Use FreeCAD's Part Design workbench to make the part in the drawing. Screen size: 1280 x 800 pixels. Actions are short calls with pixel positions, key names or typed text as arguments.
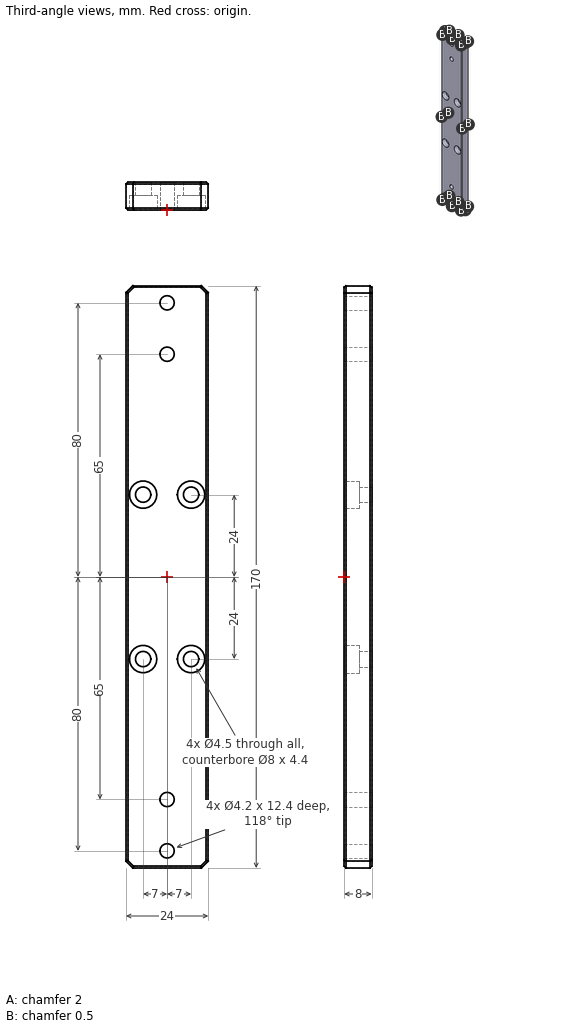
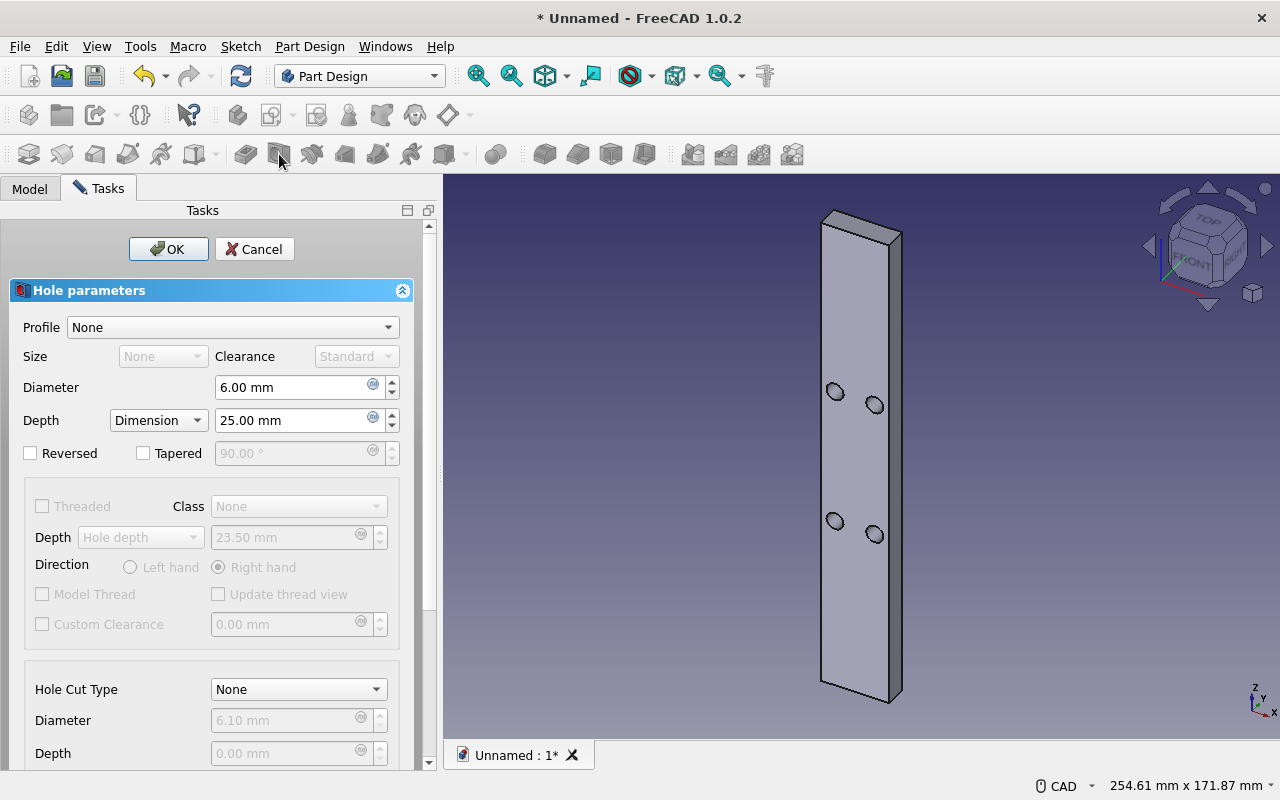
triple_click(300, 388)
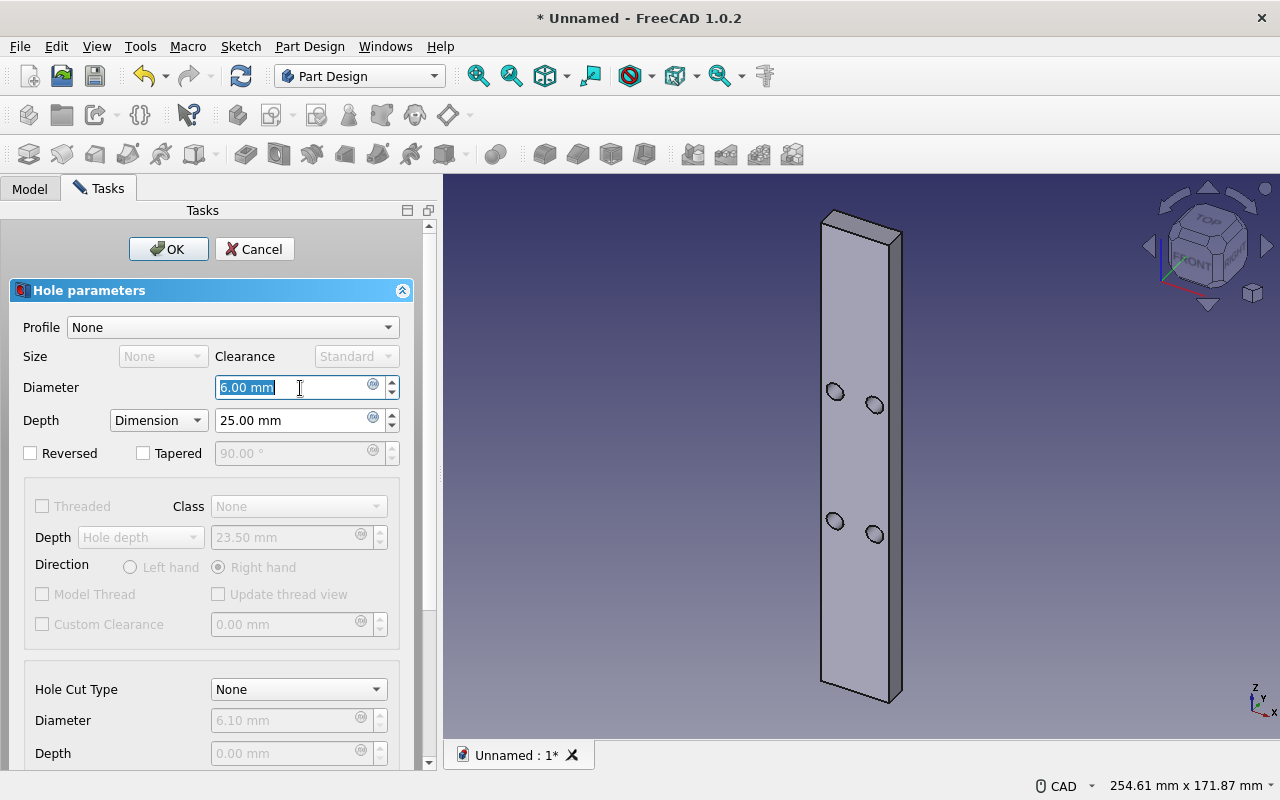
text(4.5)
key(Tab)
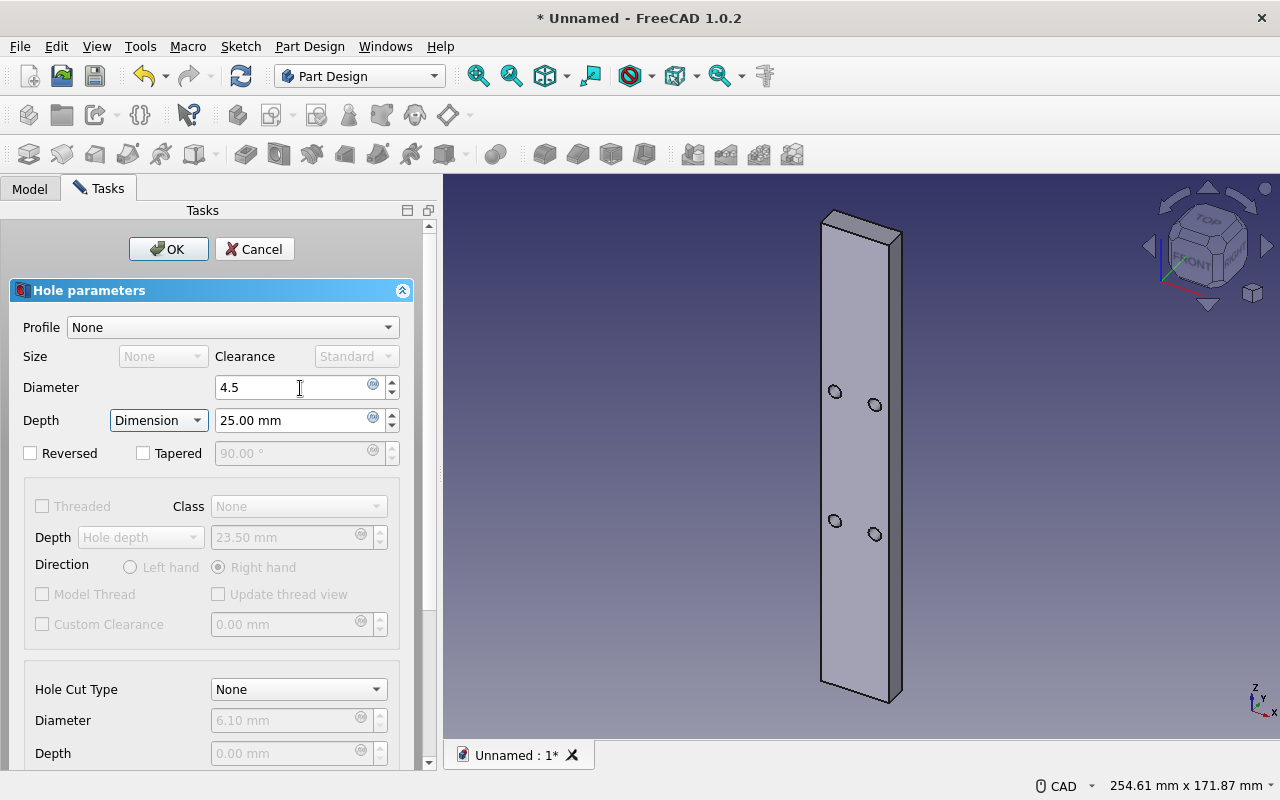
click(160, 420)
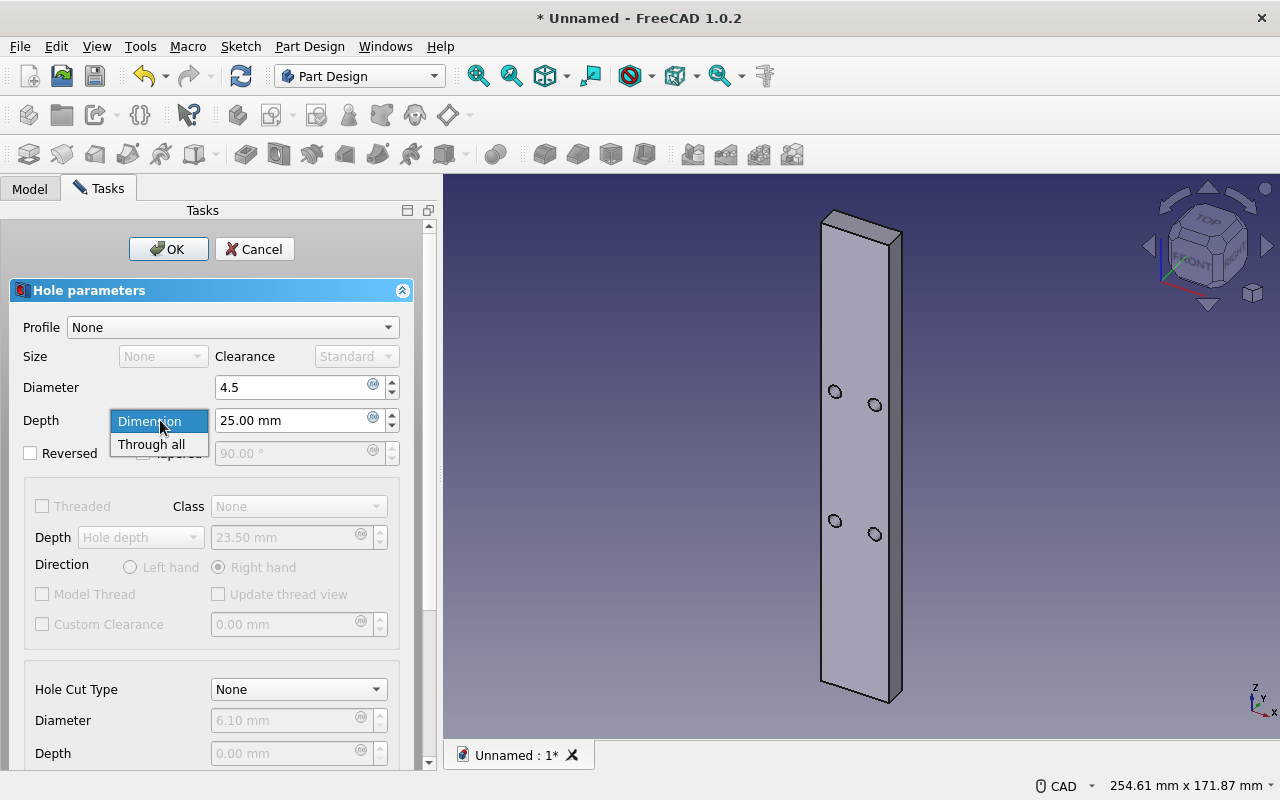
click(158, 444)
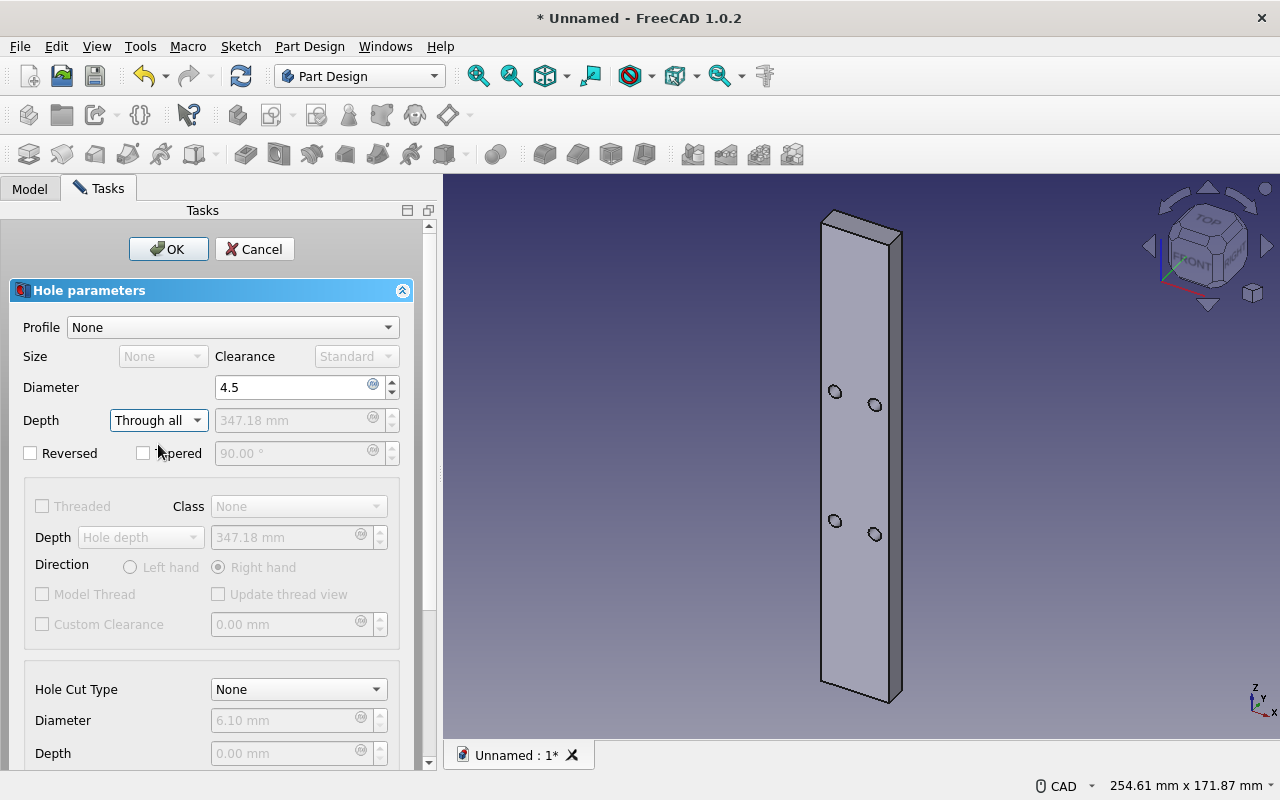
click(300, 690)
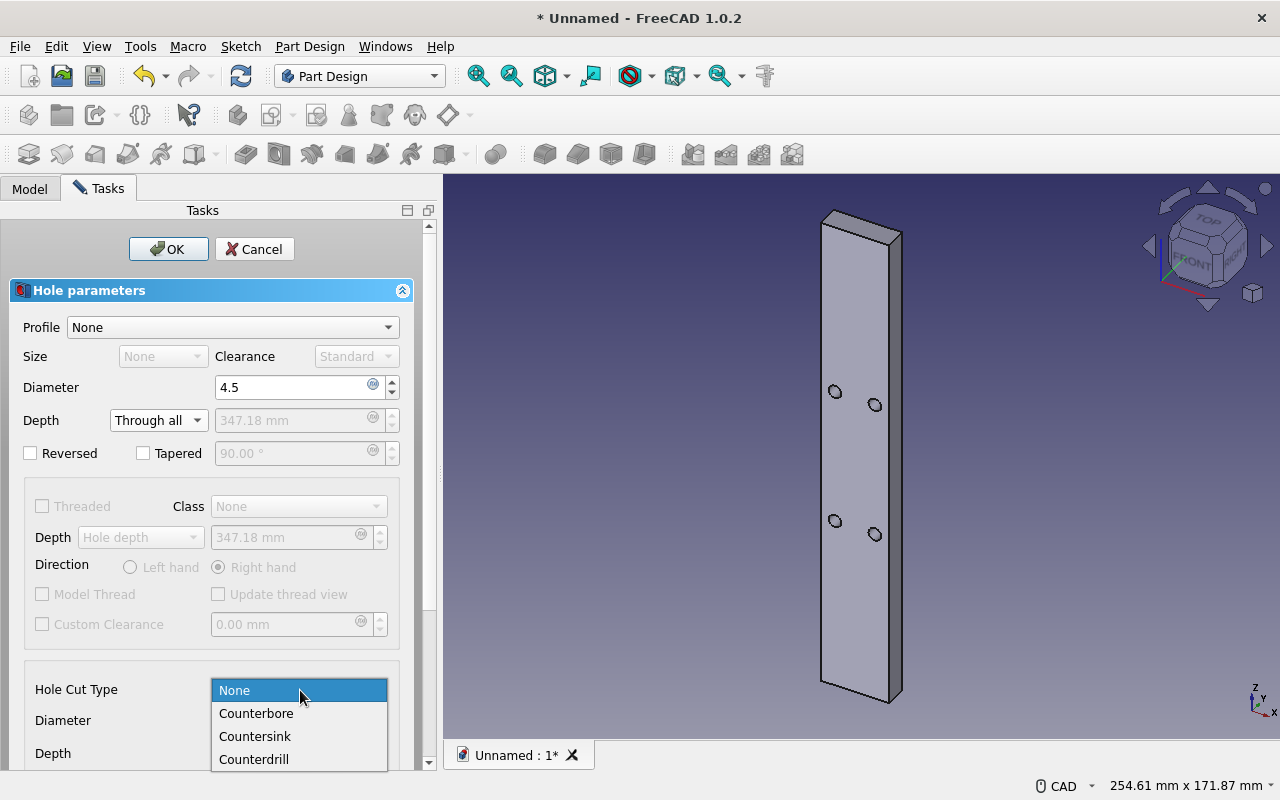
click(298, 714)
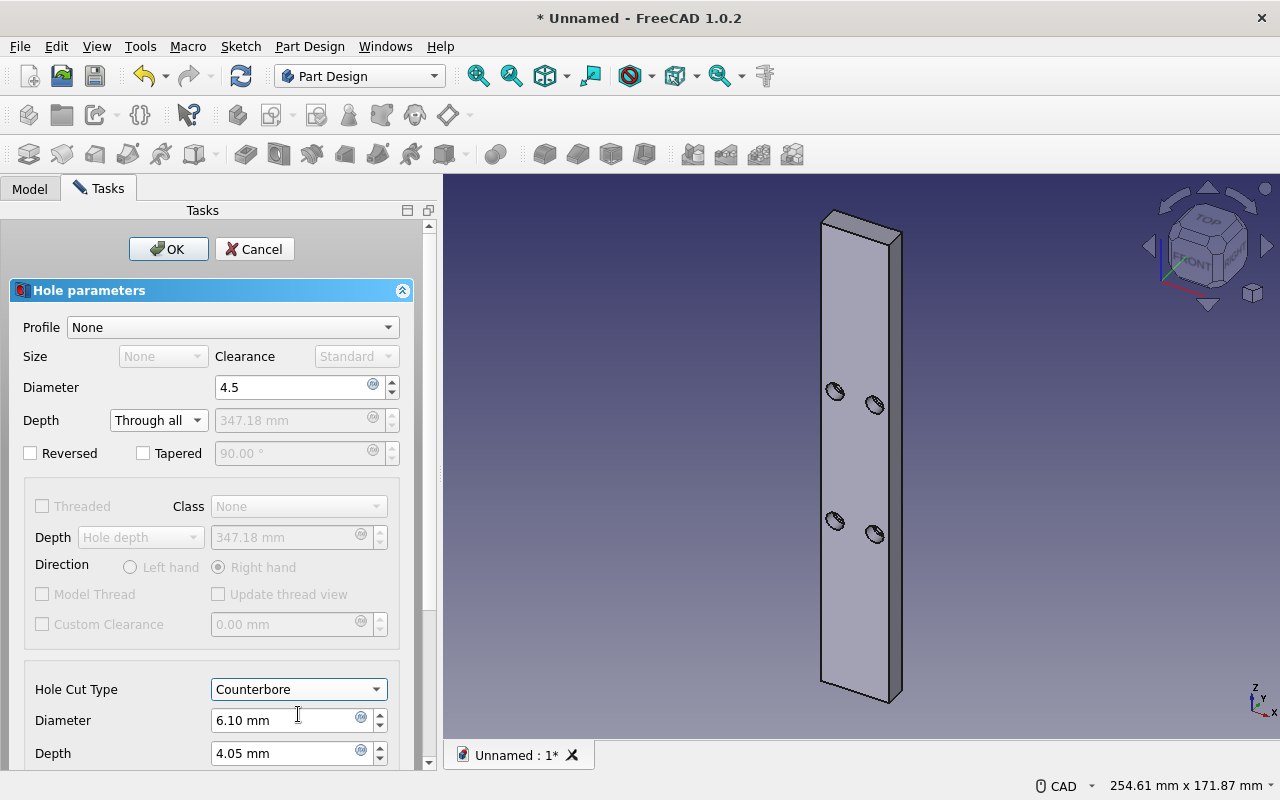
triple_click(292, 720)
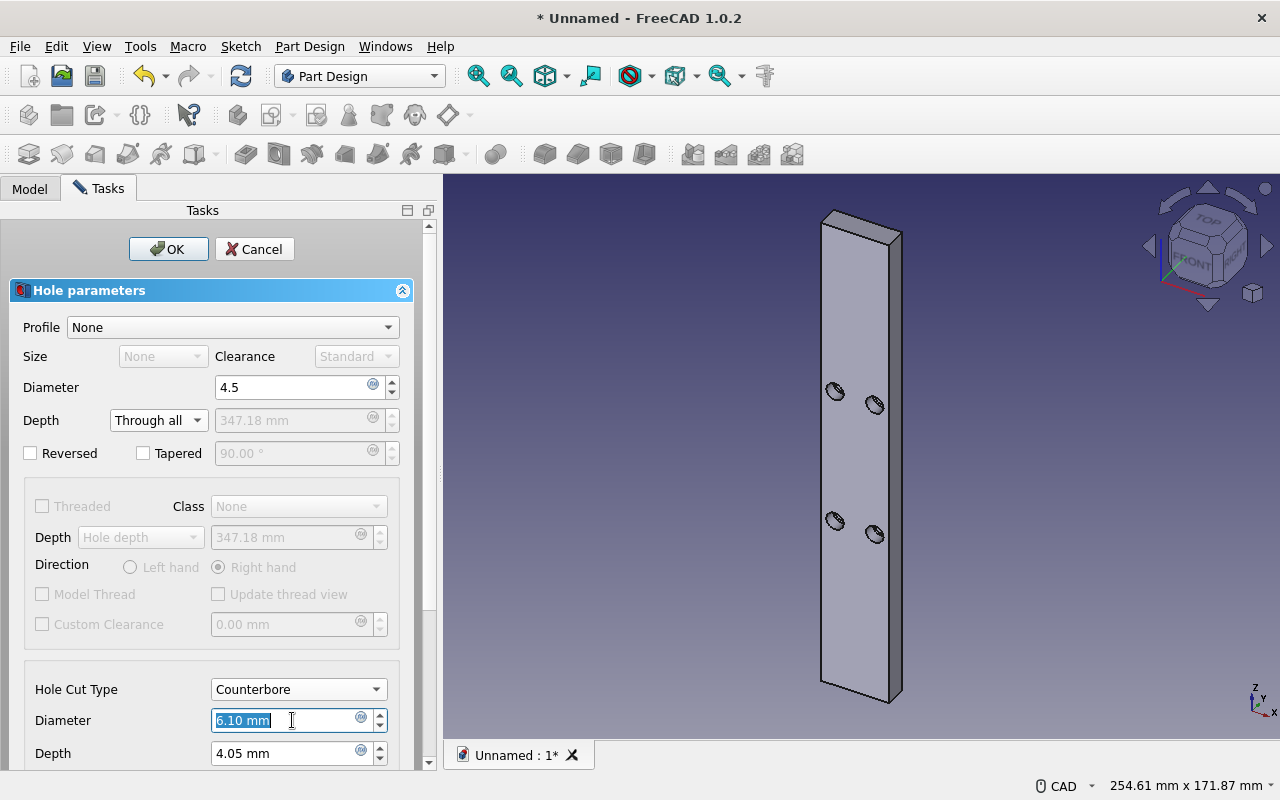
text(8)
key(Tab)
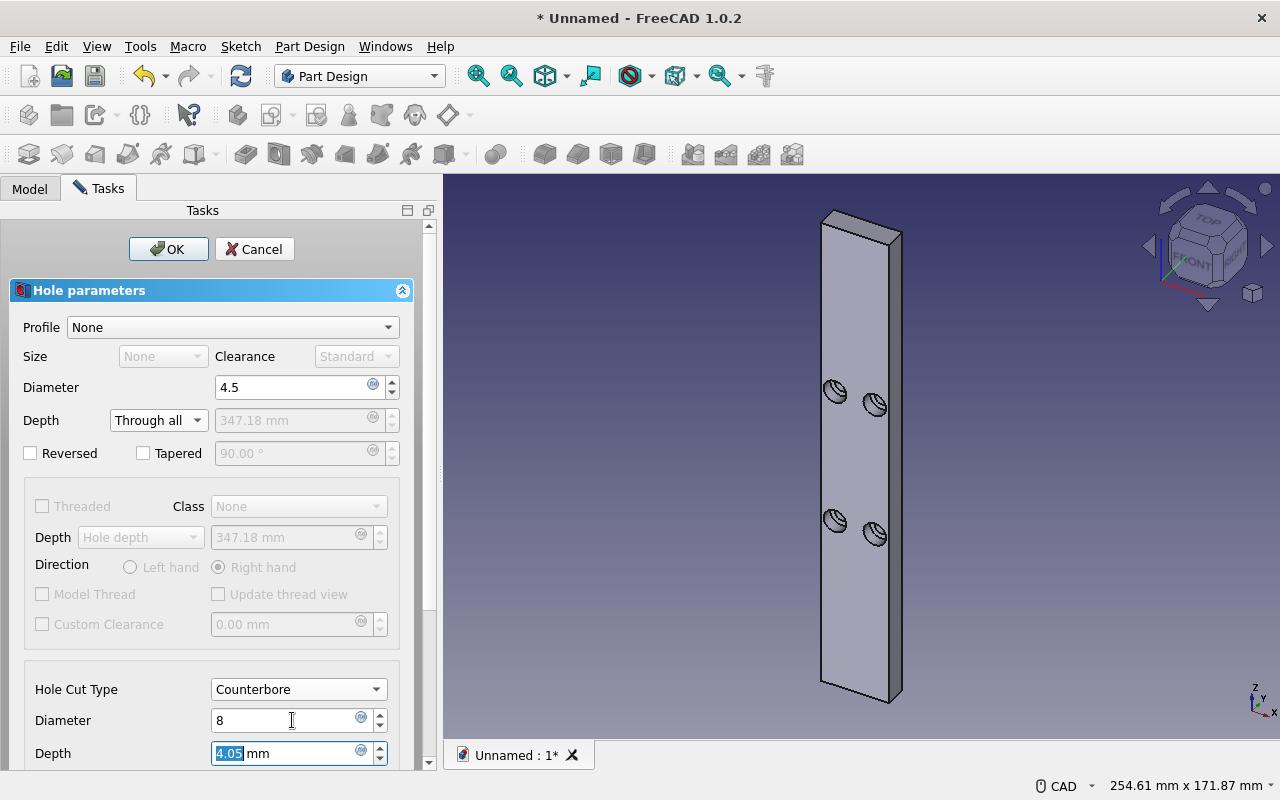
text(4.4)
key(Tab)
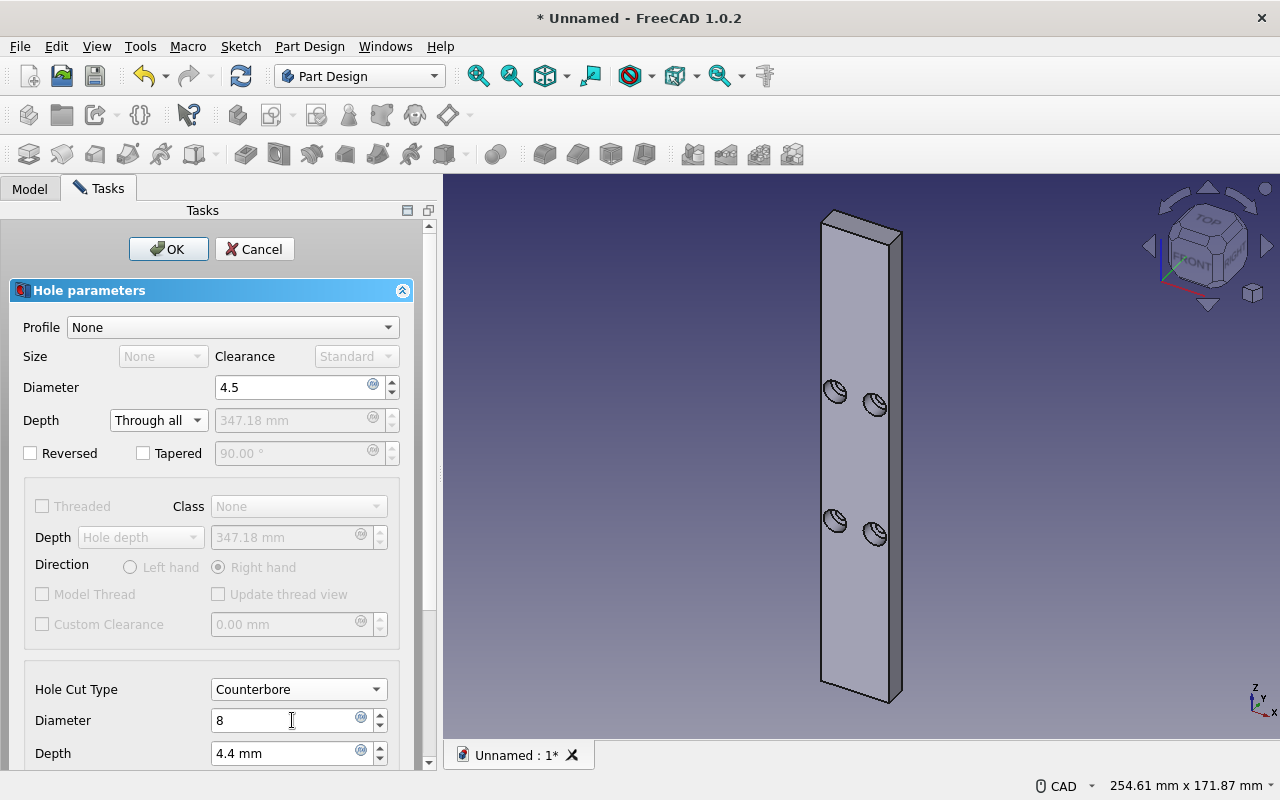
click(169, 249)